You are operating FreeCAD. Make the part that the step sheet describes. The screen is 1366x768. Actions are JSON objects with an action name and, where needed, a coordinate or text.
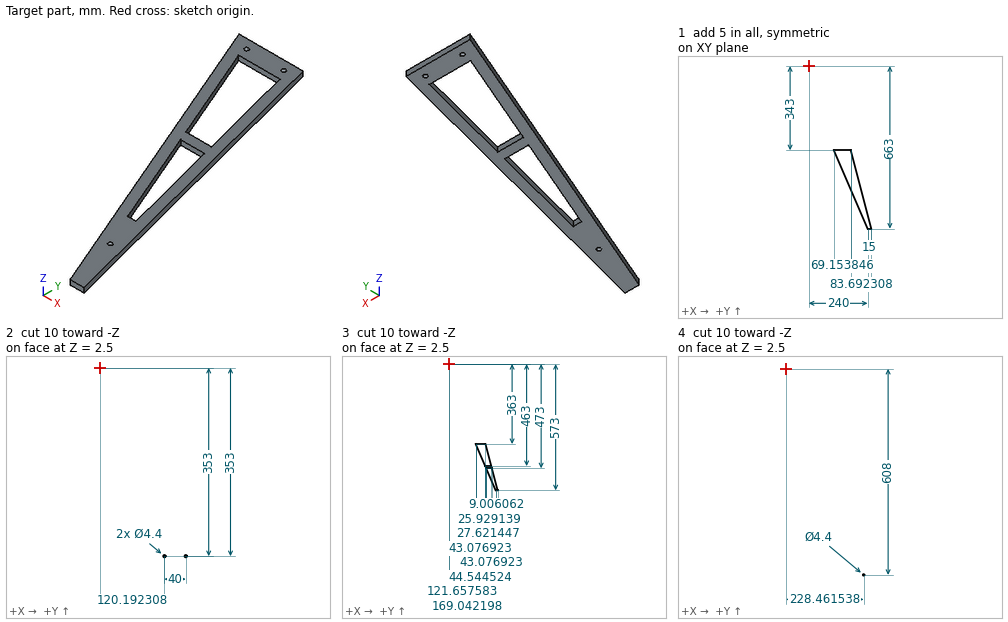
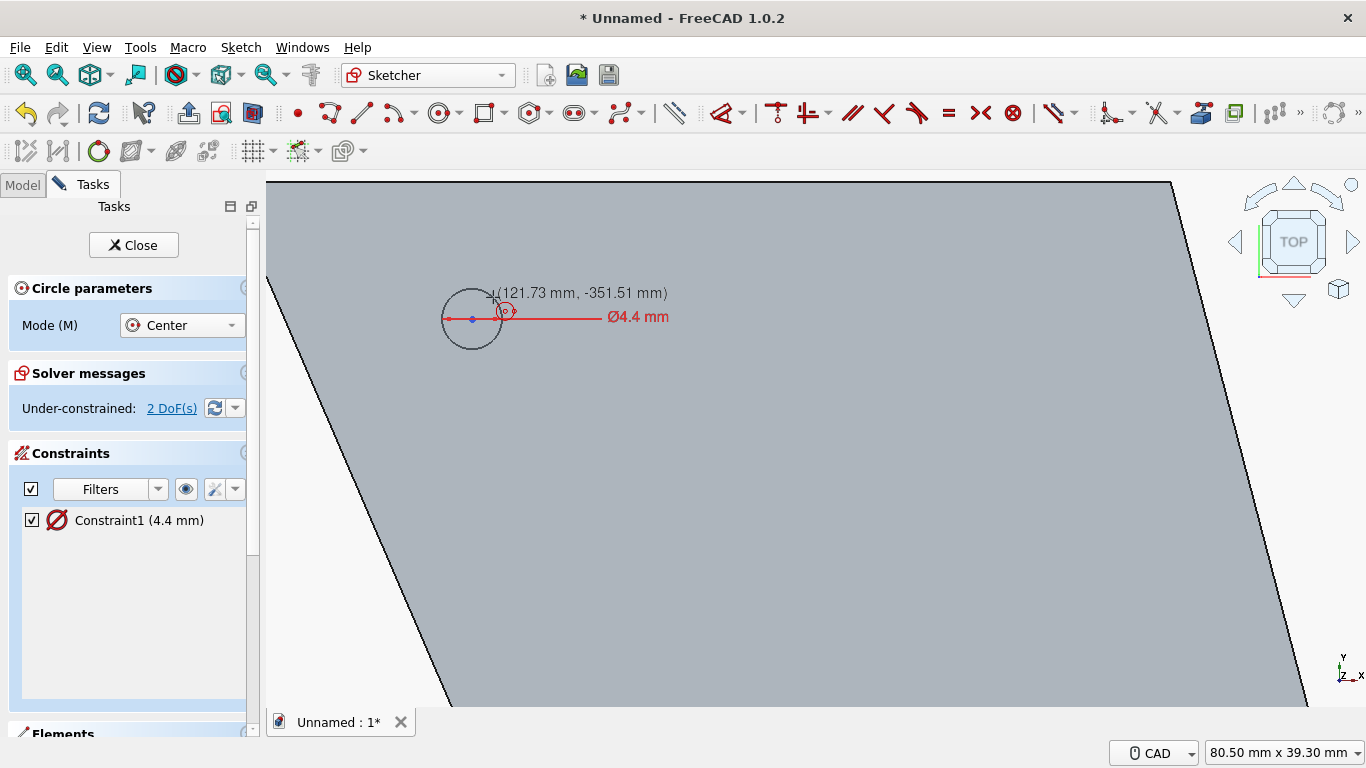
{"action": "left_click", "coordinate": [1019, 318]}
{"action": "mouse_move", "coordinate": [1040, 297]}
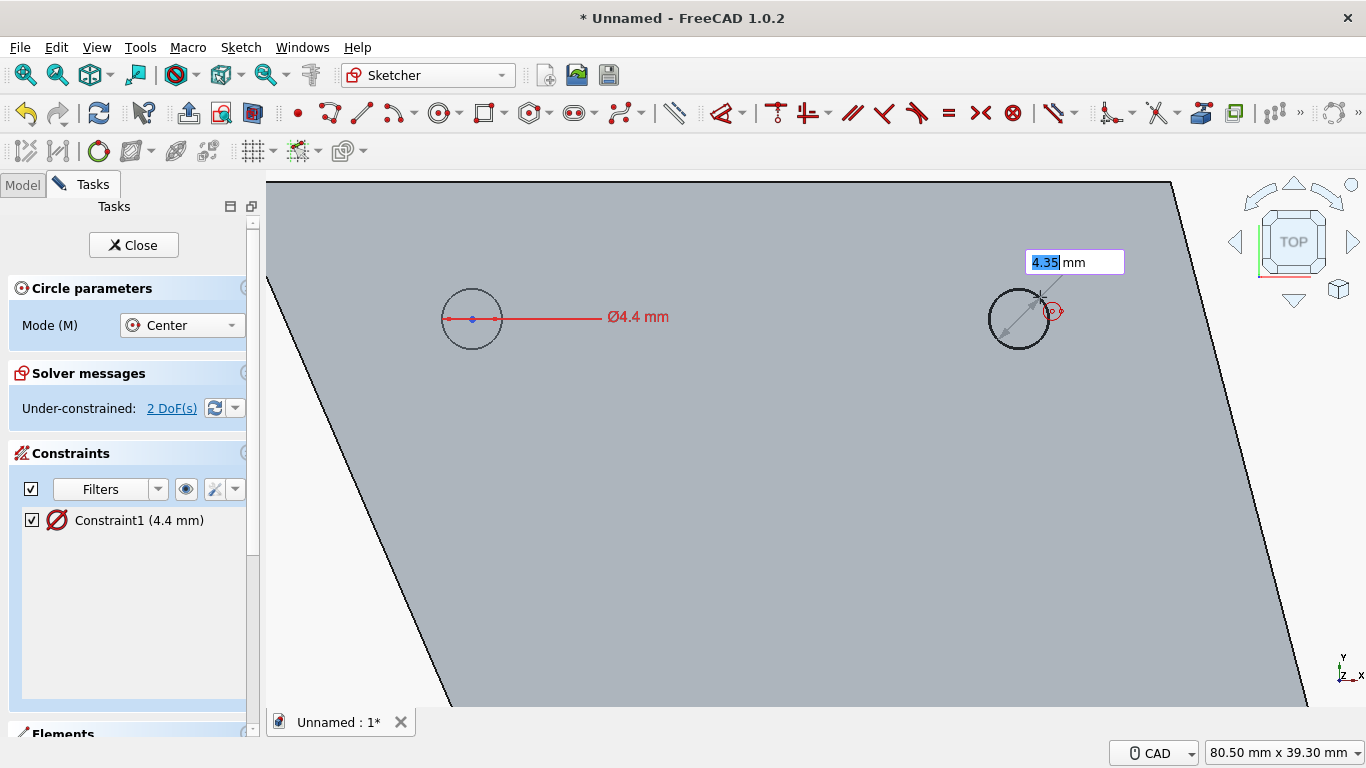
{"action": "type", "text": "4.4"}
{"action": "key", "text": "Return"}
{"action": "key", "text": "Escape"}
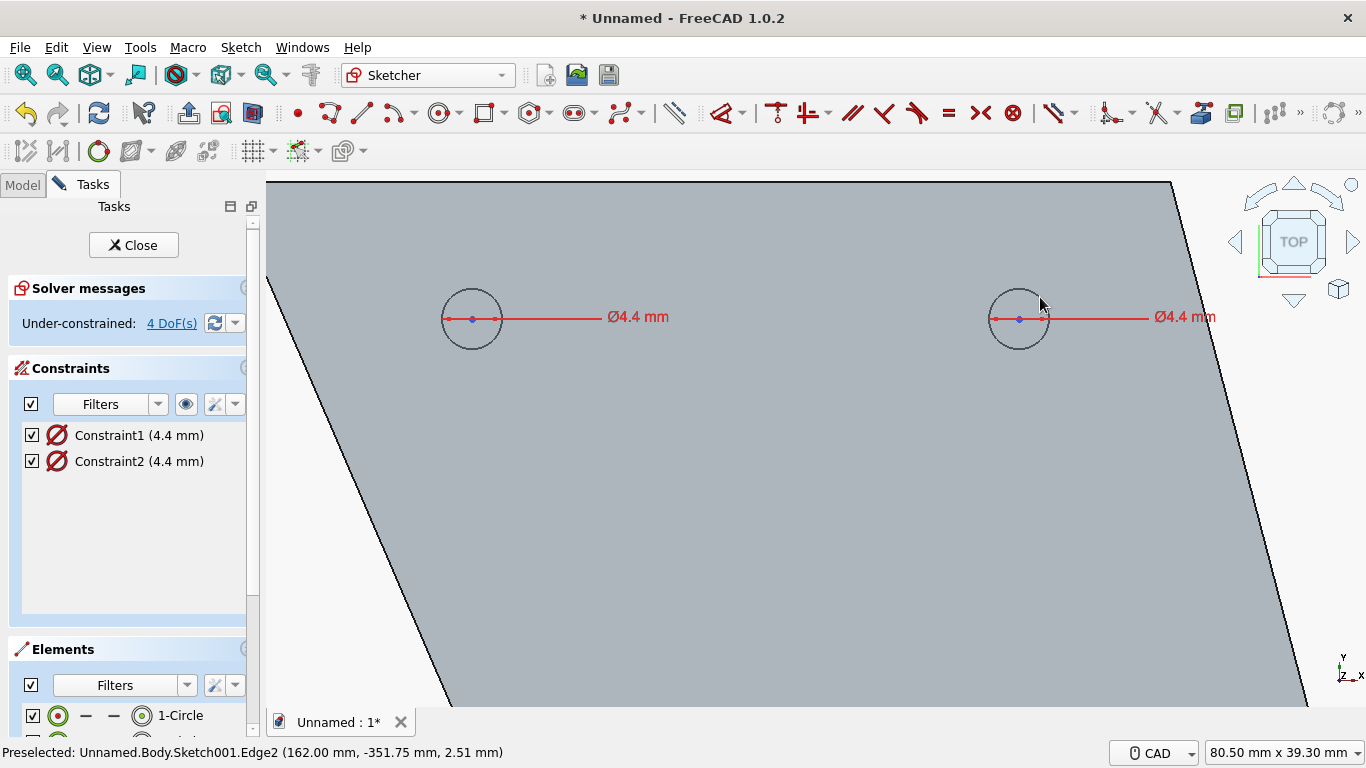
{"action": "key", "text": "d"}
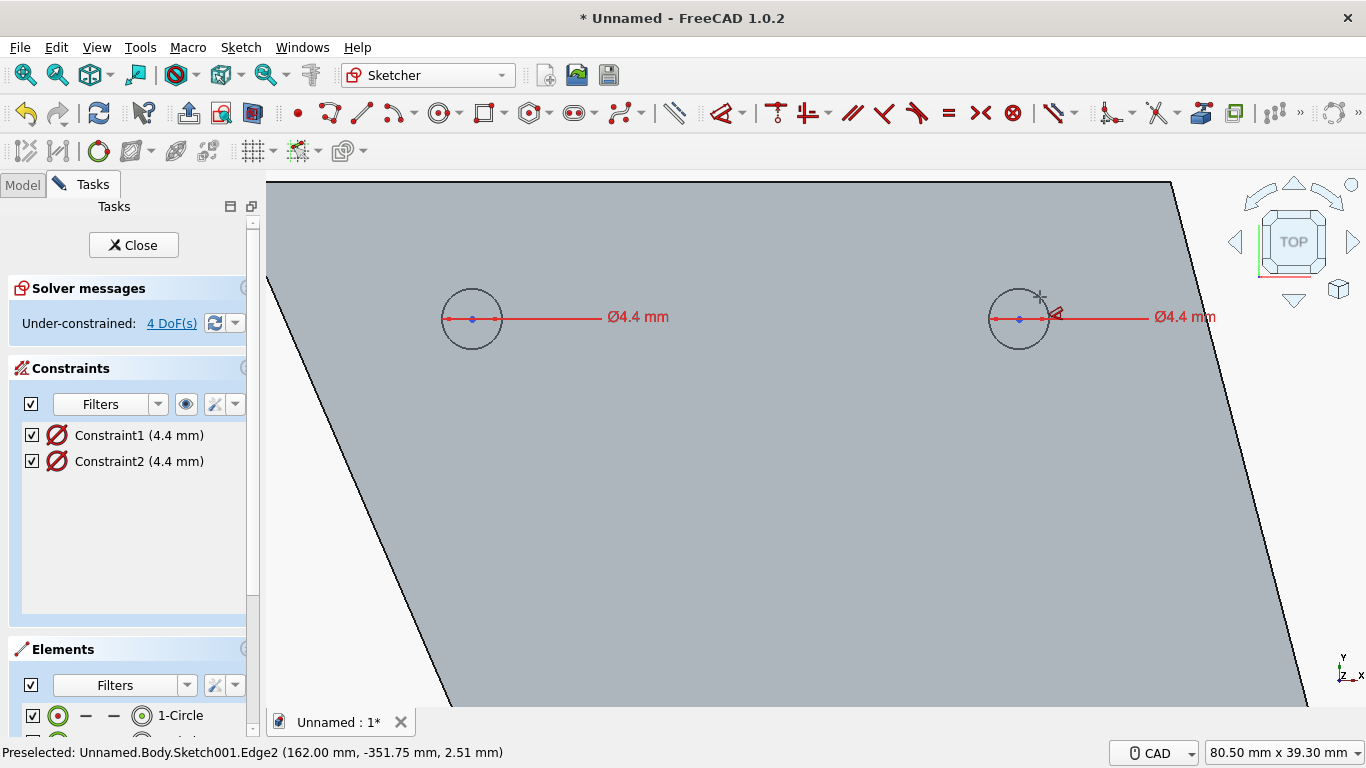
{"action": "left_click", "coordinate": [472, 319]}
{"action": "left_click", "coordinate": [506, 258]}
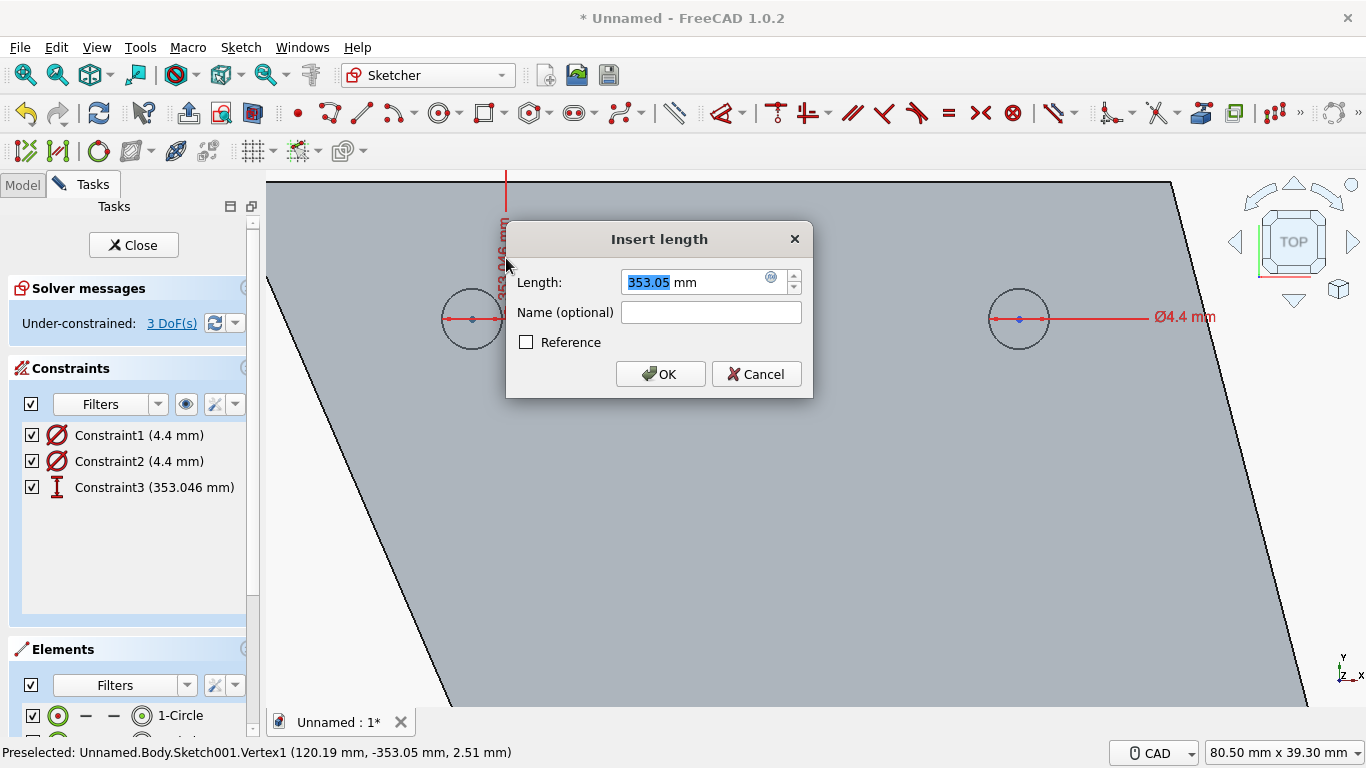
{"action": "type", "text": "353"}
{"action": "key", "text": "Return"}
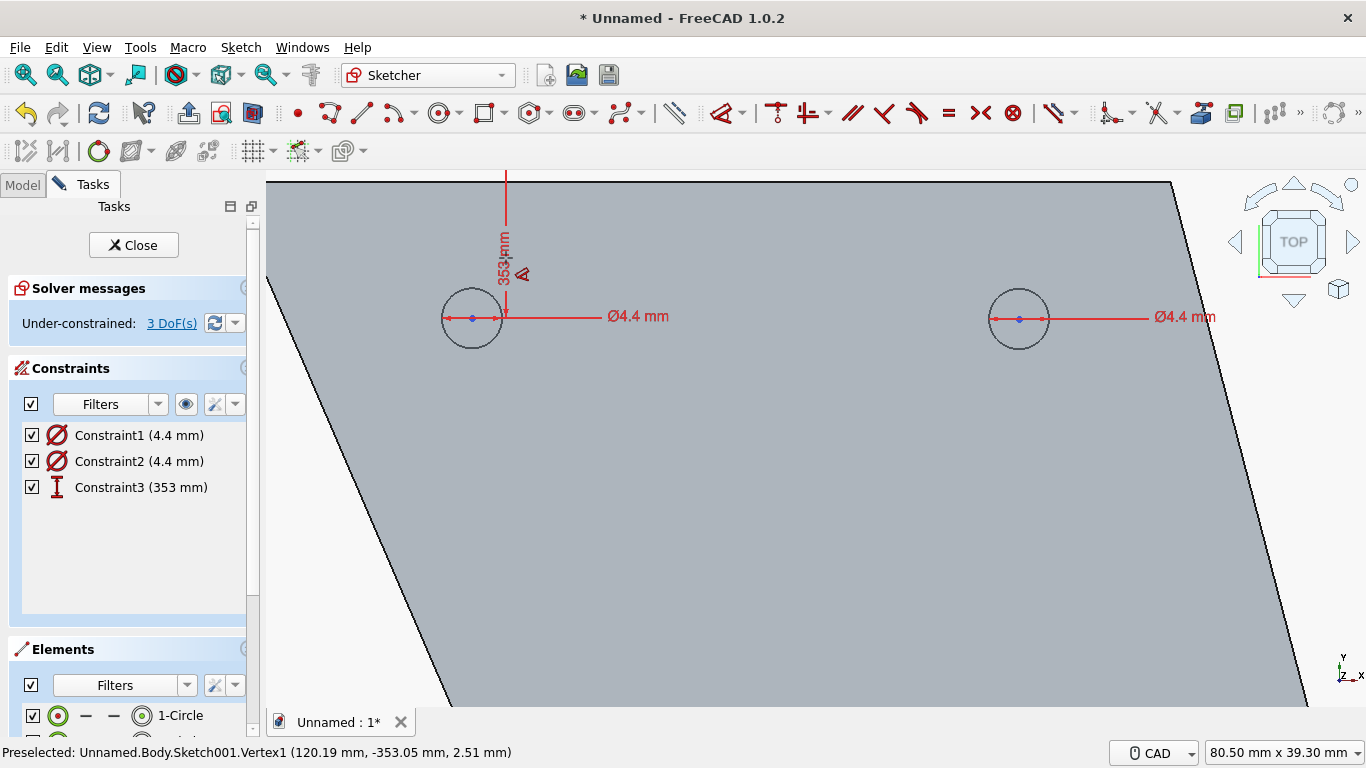
{"action": "left_click", "coordinate": [1019, 319]}
{"action": "left_click", "coordinate": [1053, 258]}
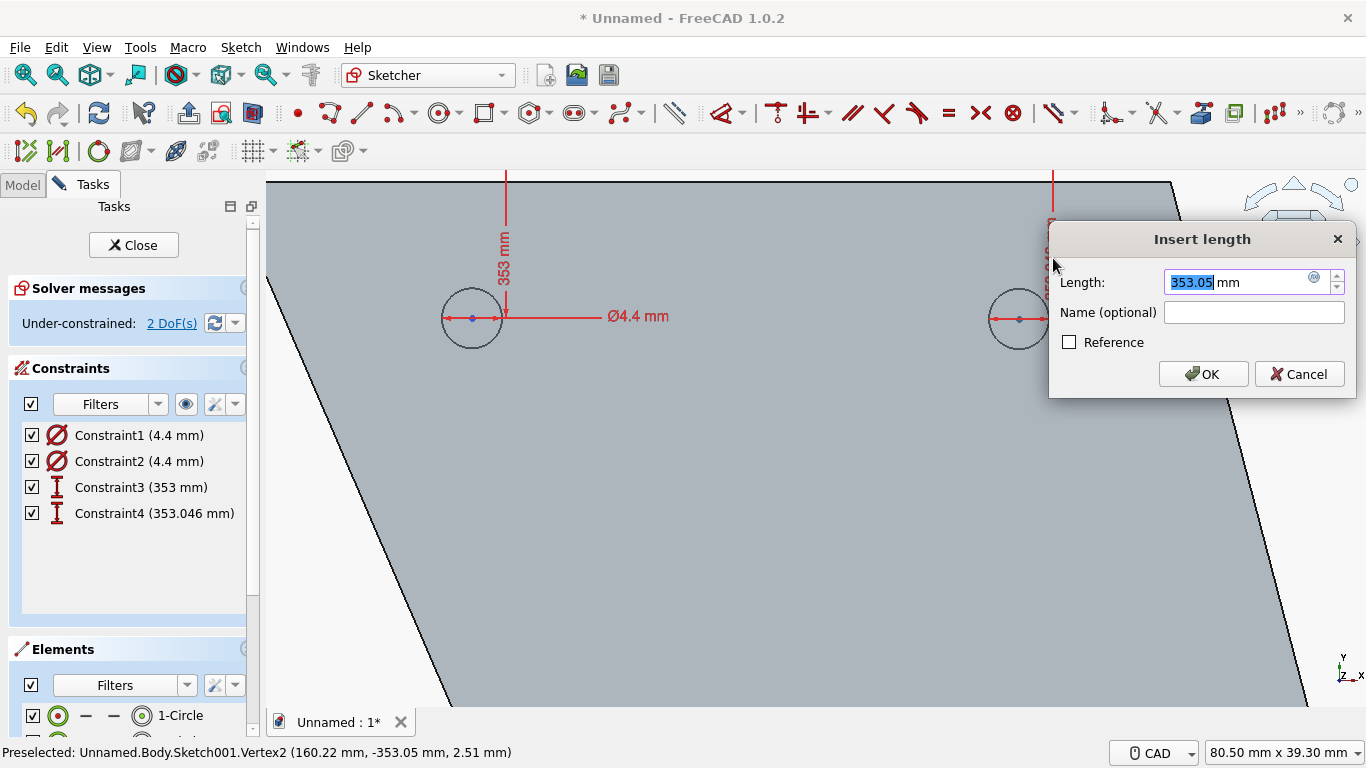
{"action": "type", "text": "353"}
{"action": "key", "text": "Return"}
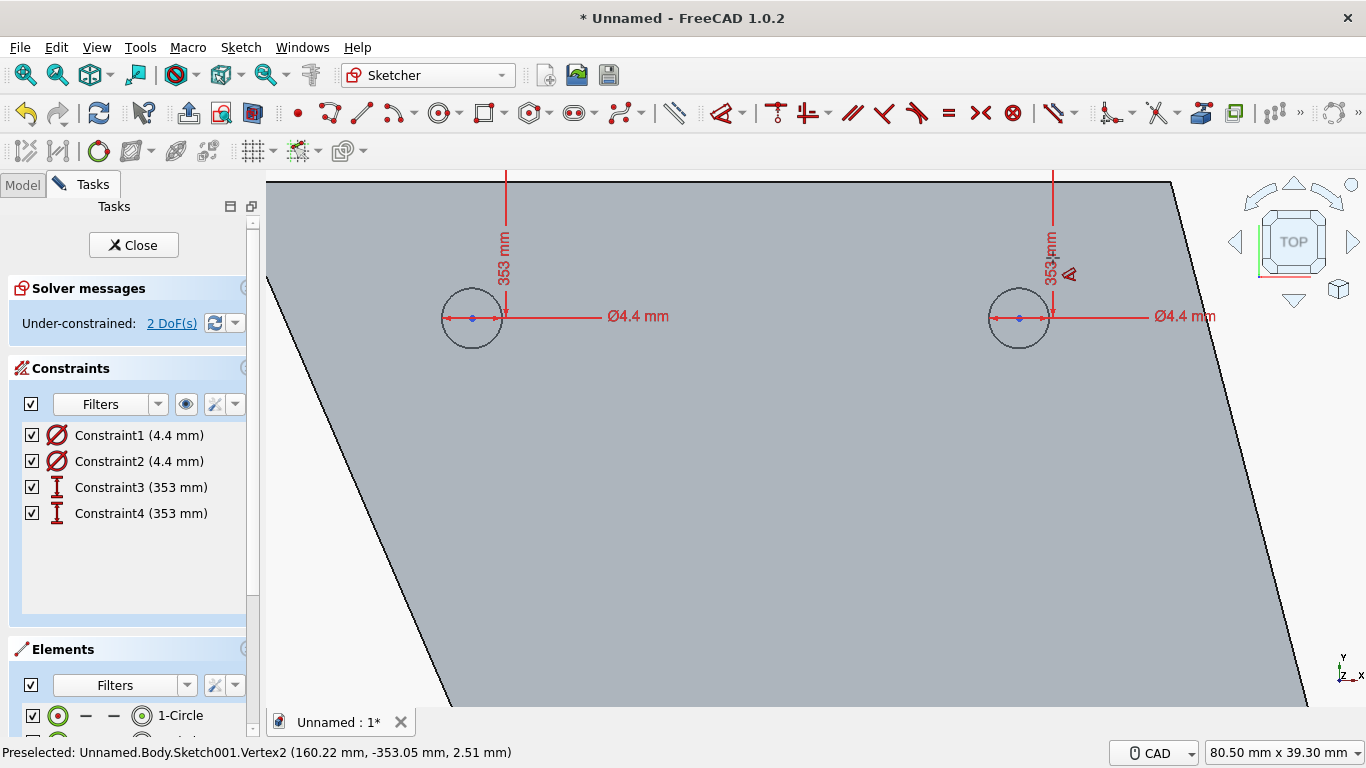
{"action": "left_click", "coordinate": [472, 318]}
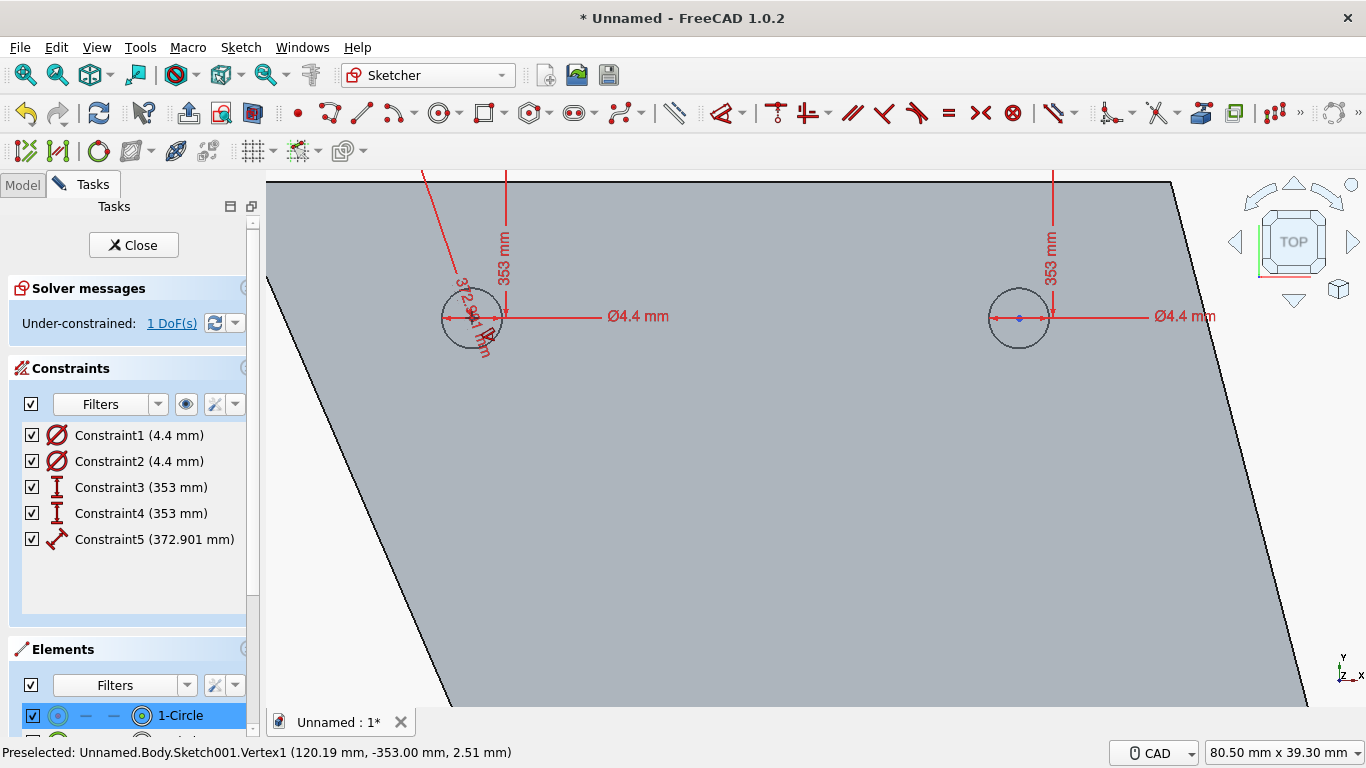
{"action": "left_click", "coordinate": [1019, 318]}
{"action": "left_click", "coordinate": [746, 352]}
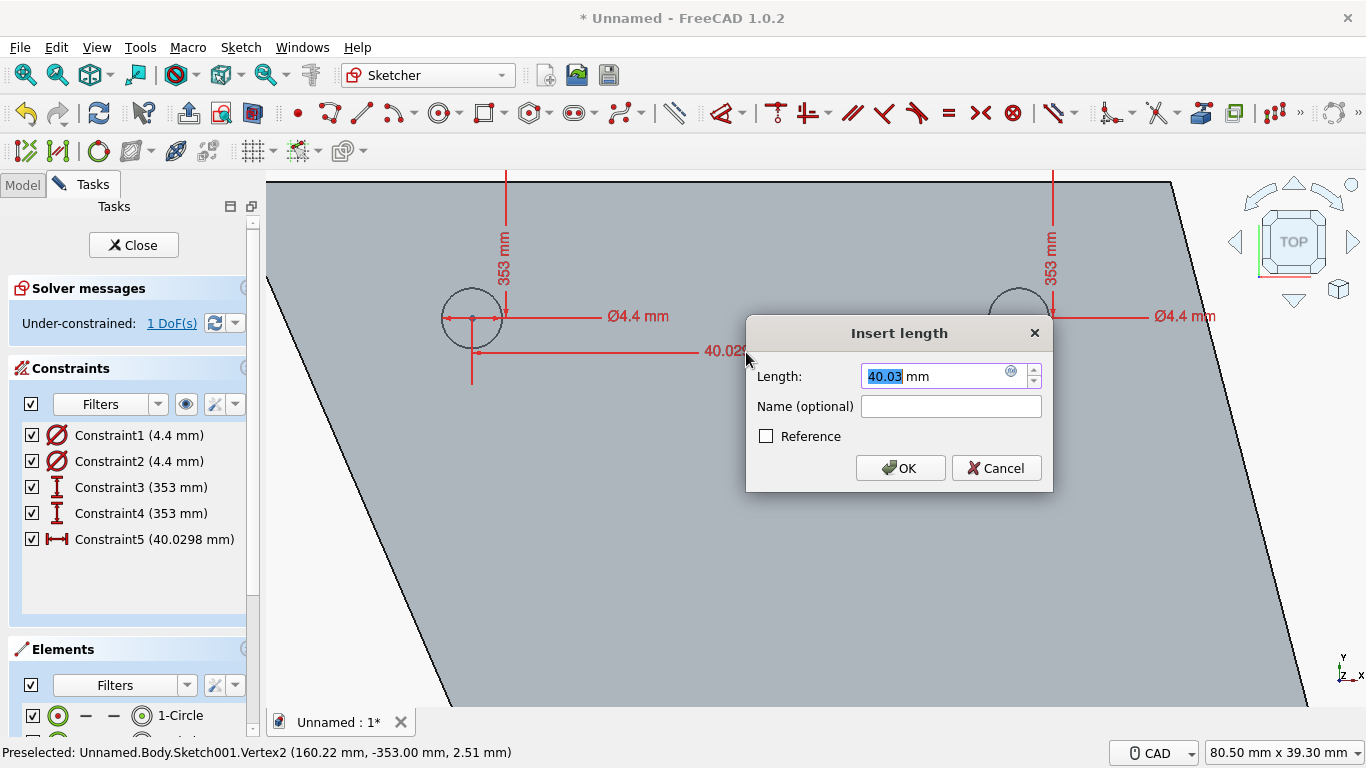
{"action": "type", "text": "40"}
{"action": "key", "text": "Return"}